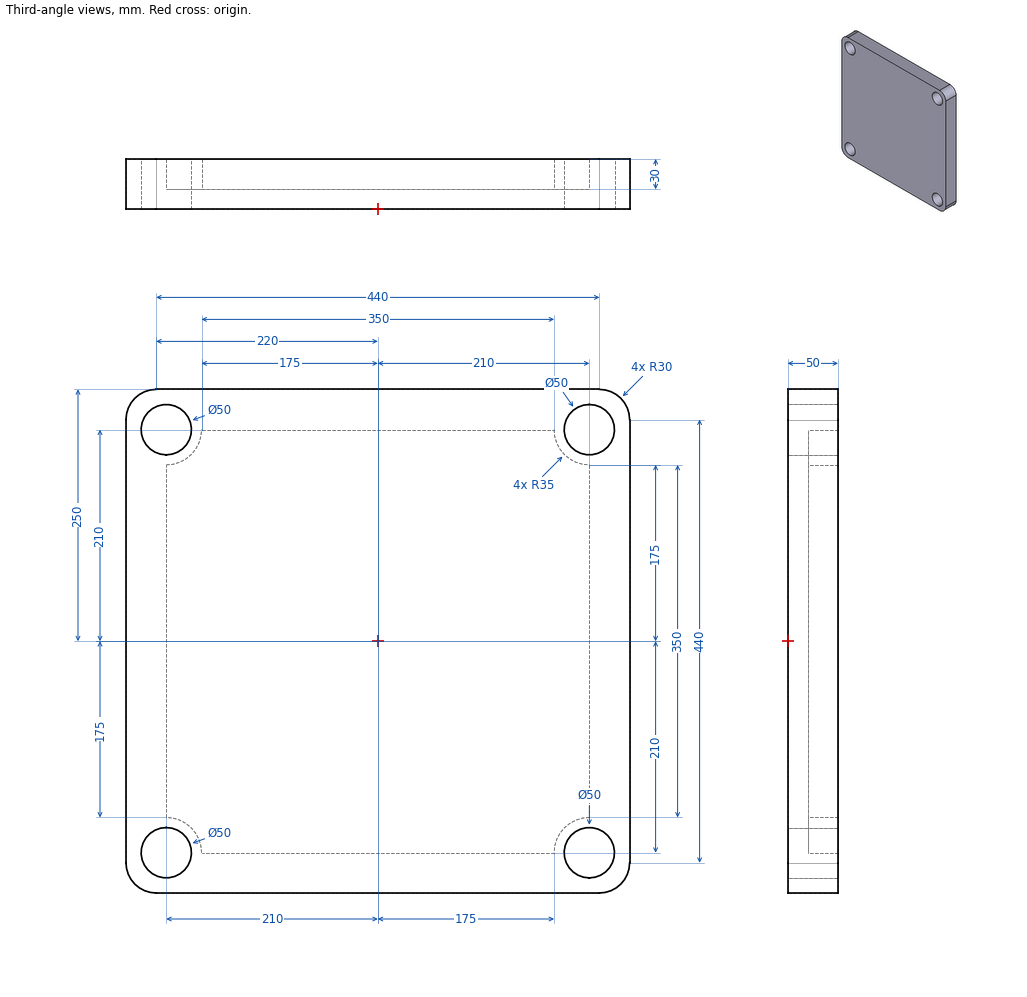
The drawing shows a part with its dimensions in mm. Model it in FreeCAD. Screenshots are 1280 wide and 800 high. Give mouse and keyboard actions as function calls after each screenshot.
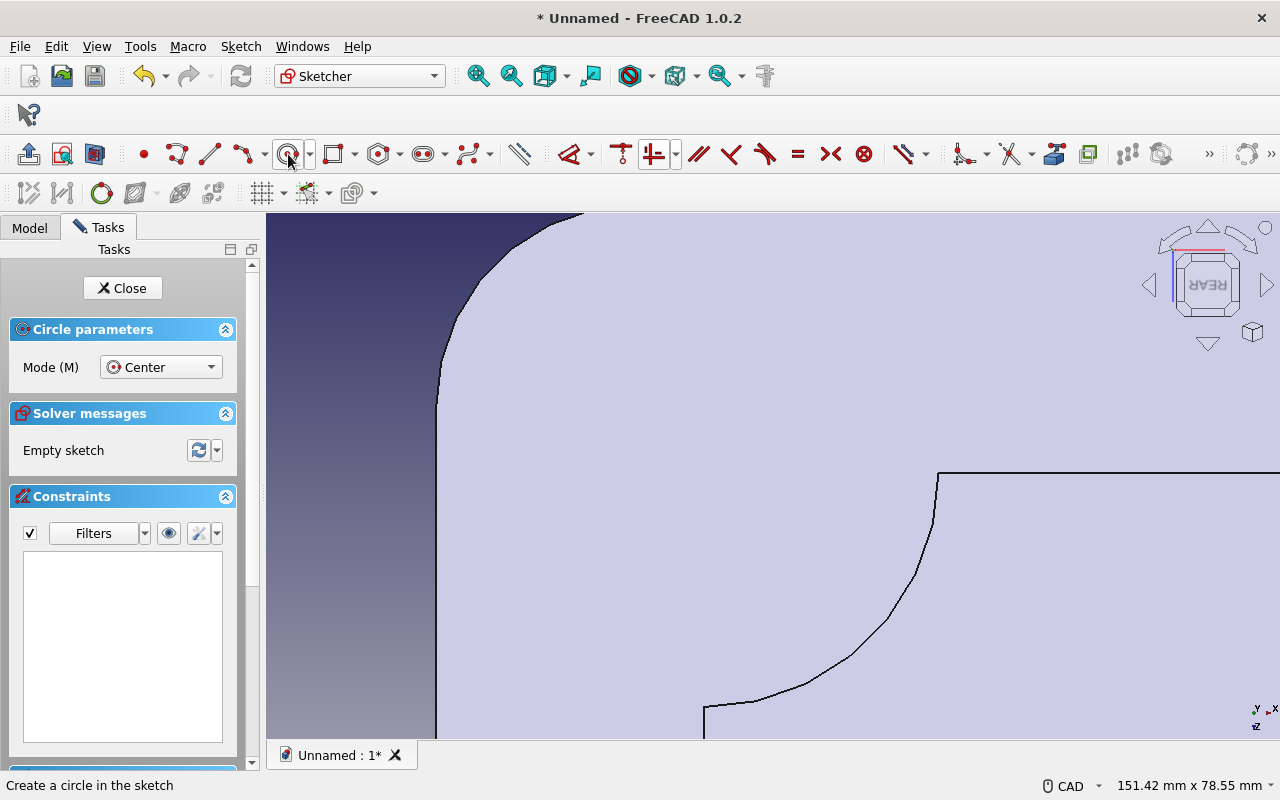
click(704, 473)
move(823, 354)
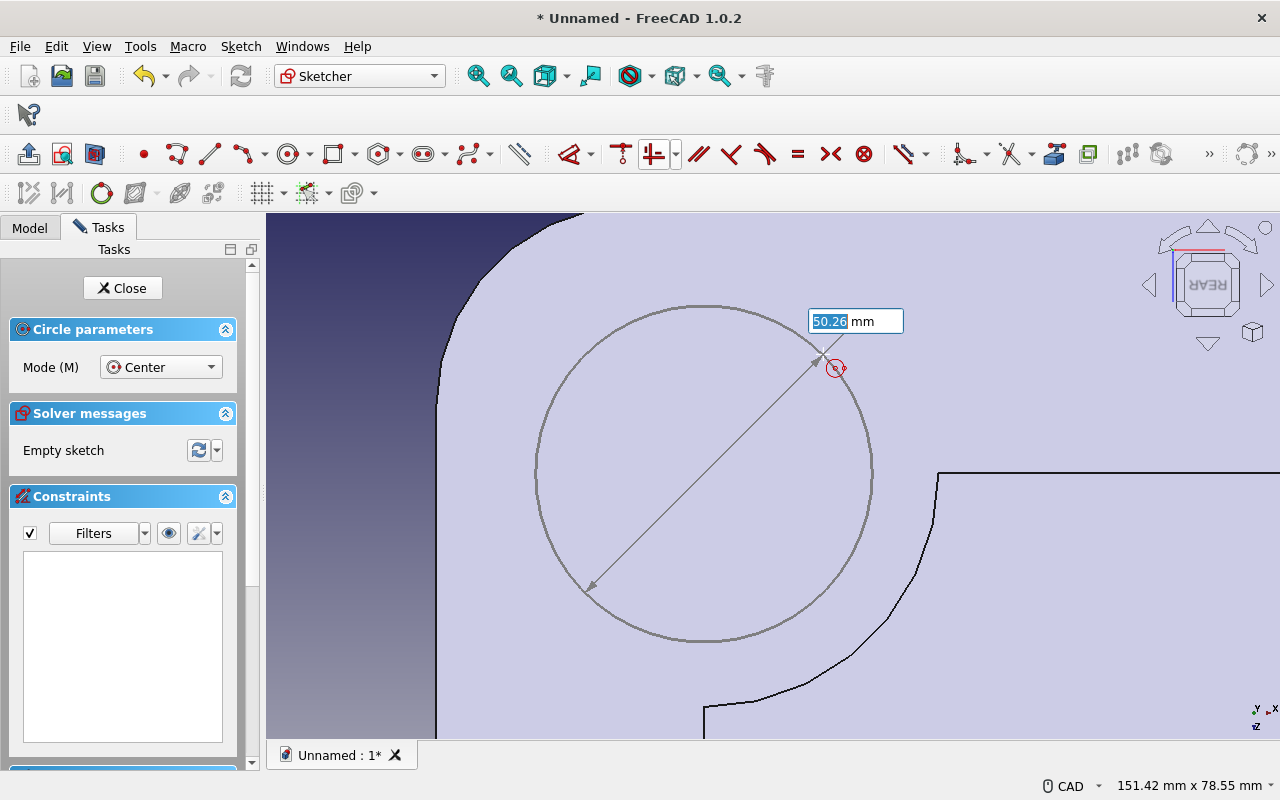
text(50)
key(Return)
key(Escape)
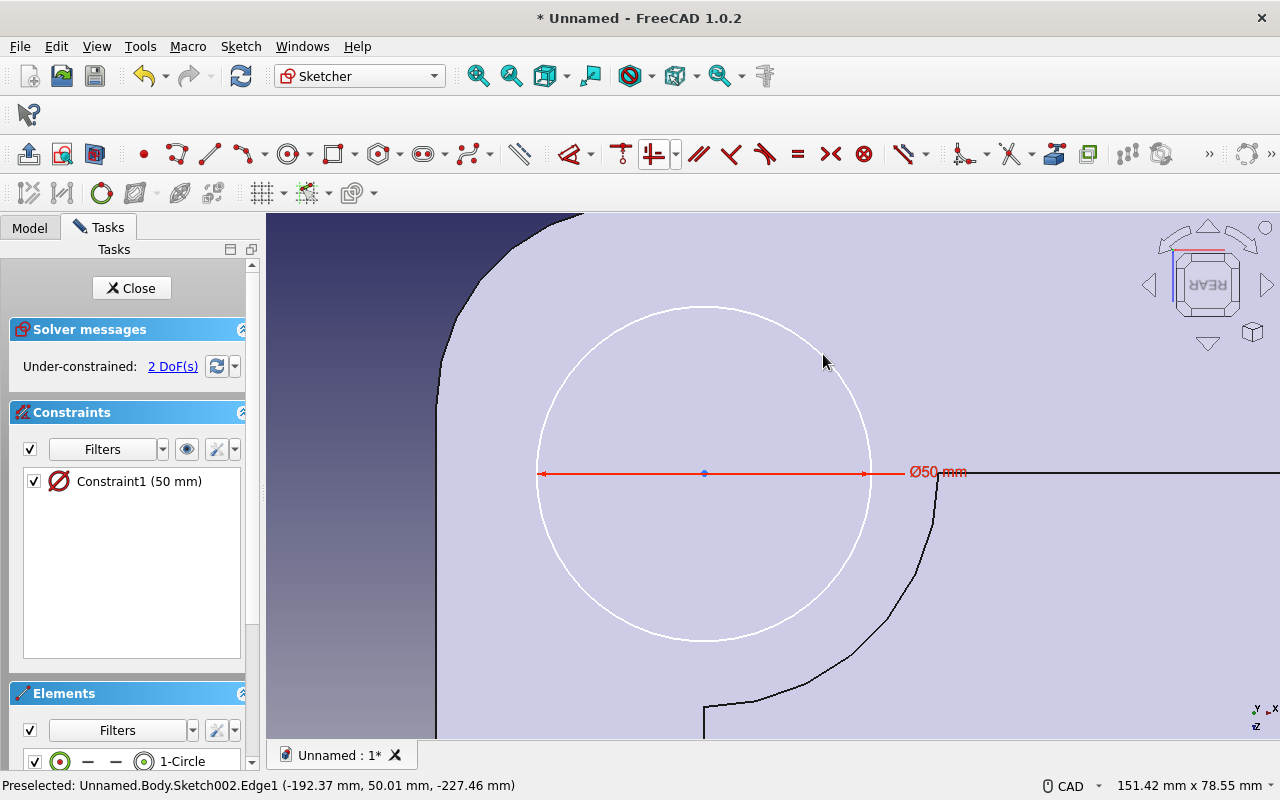
click(568, 154)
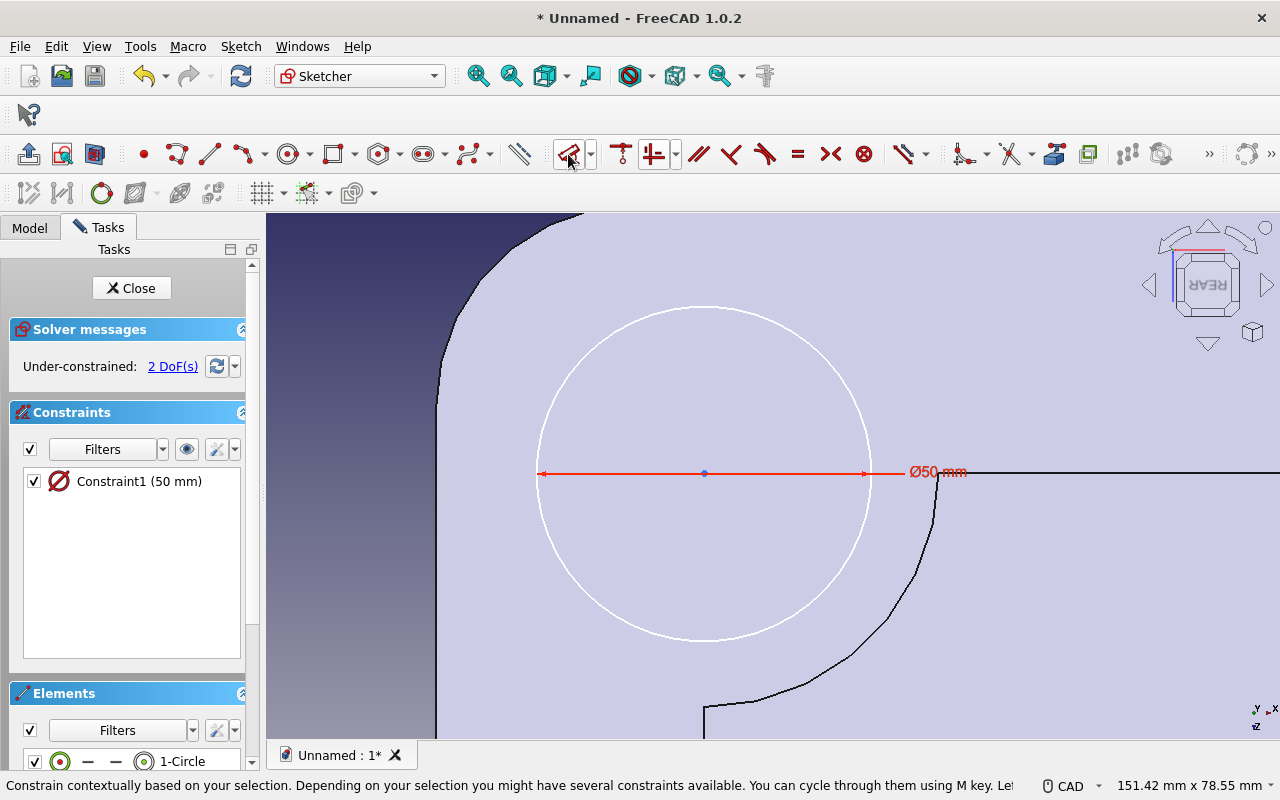
click(704, 474)
click(909, 440)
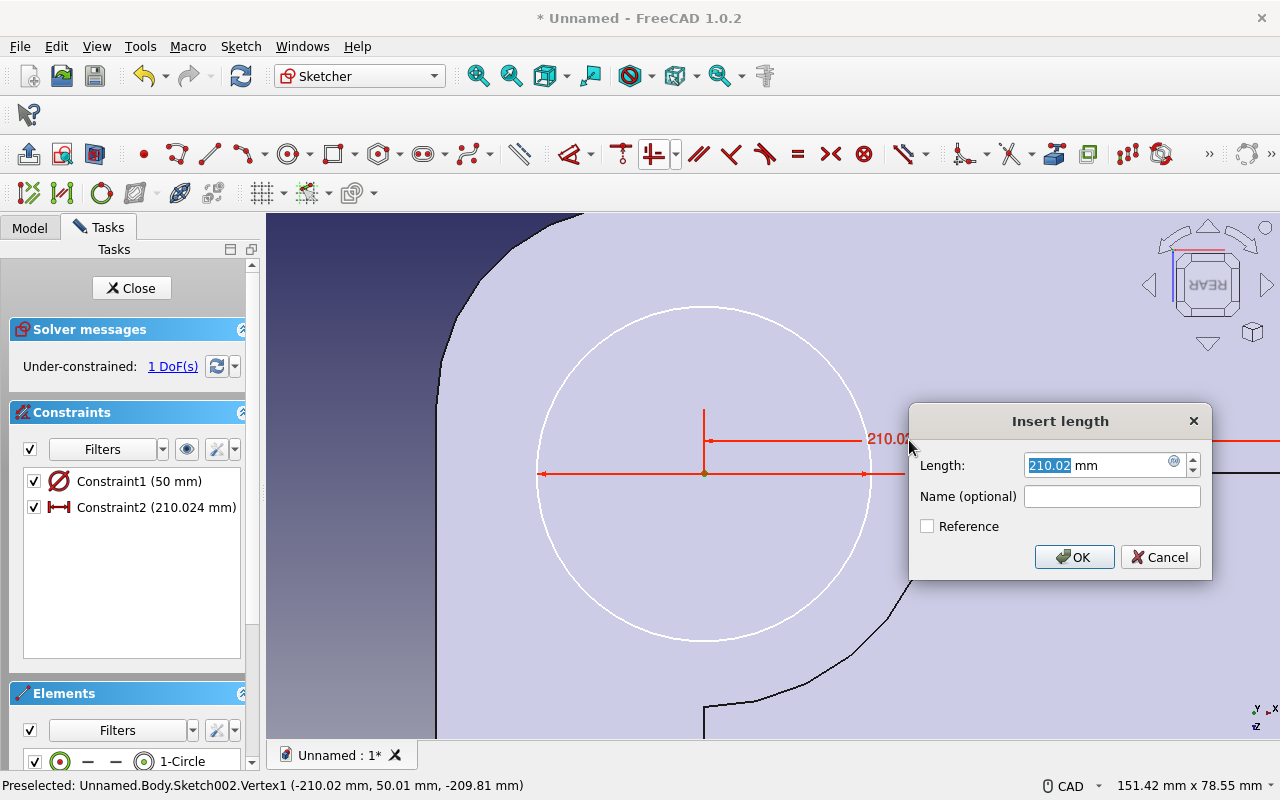
text(210)
key(Return)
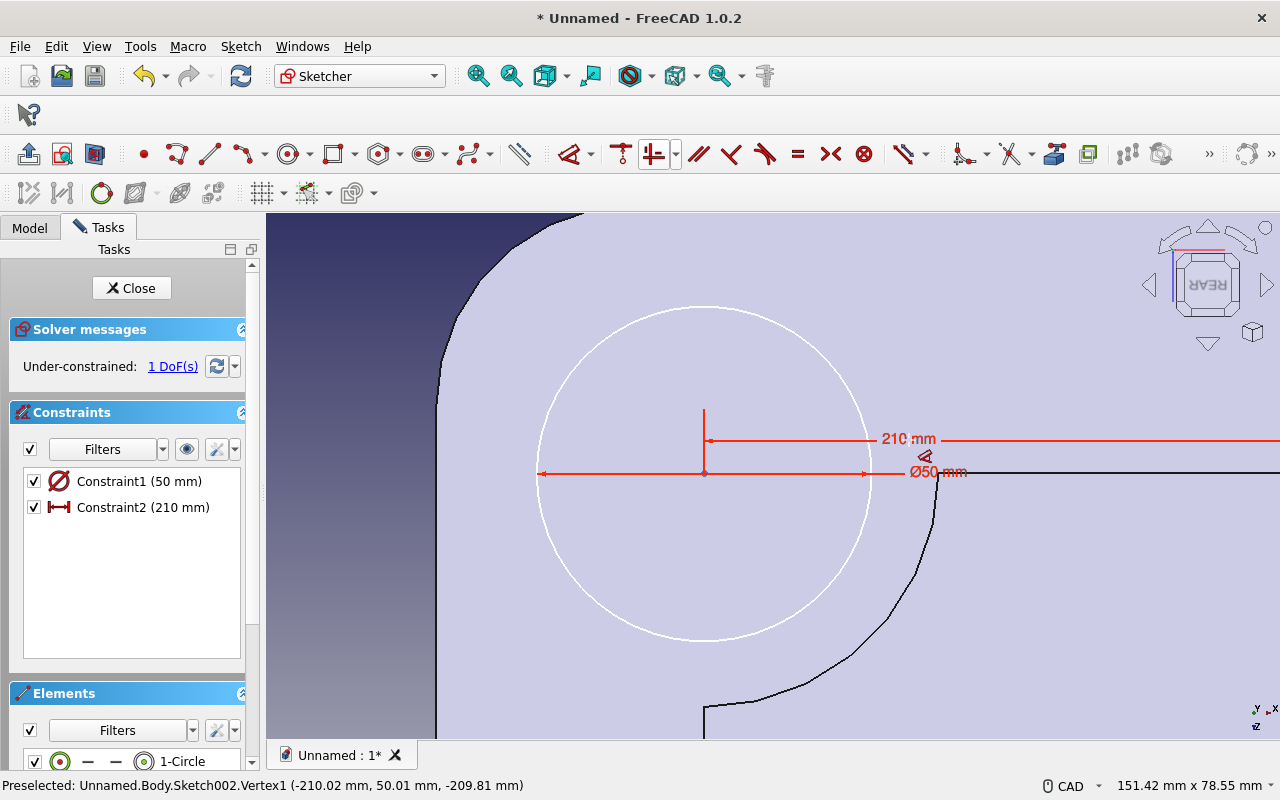
click(704, 474)
click(670, 592)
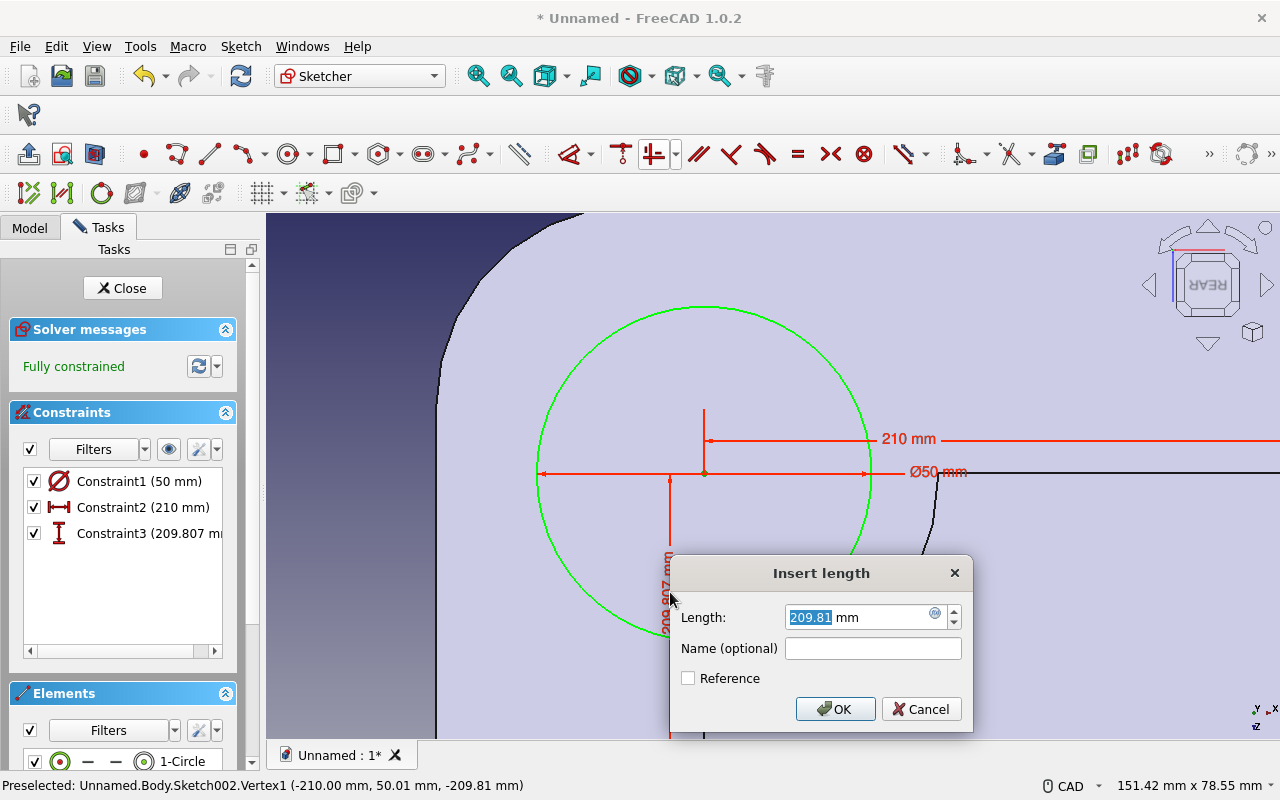
text(210)
key(Return)
key(Escape)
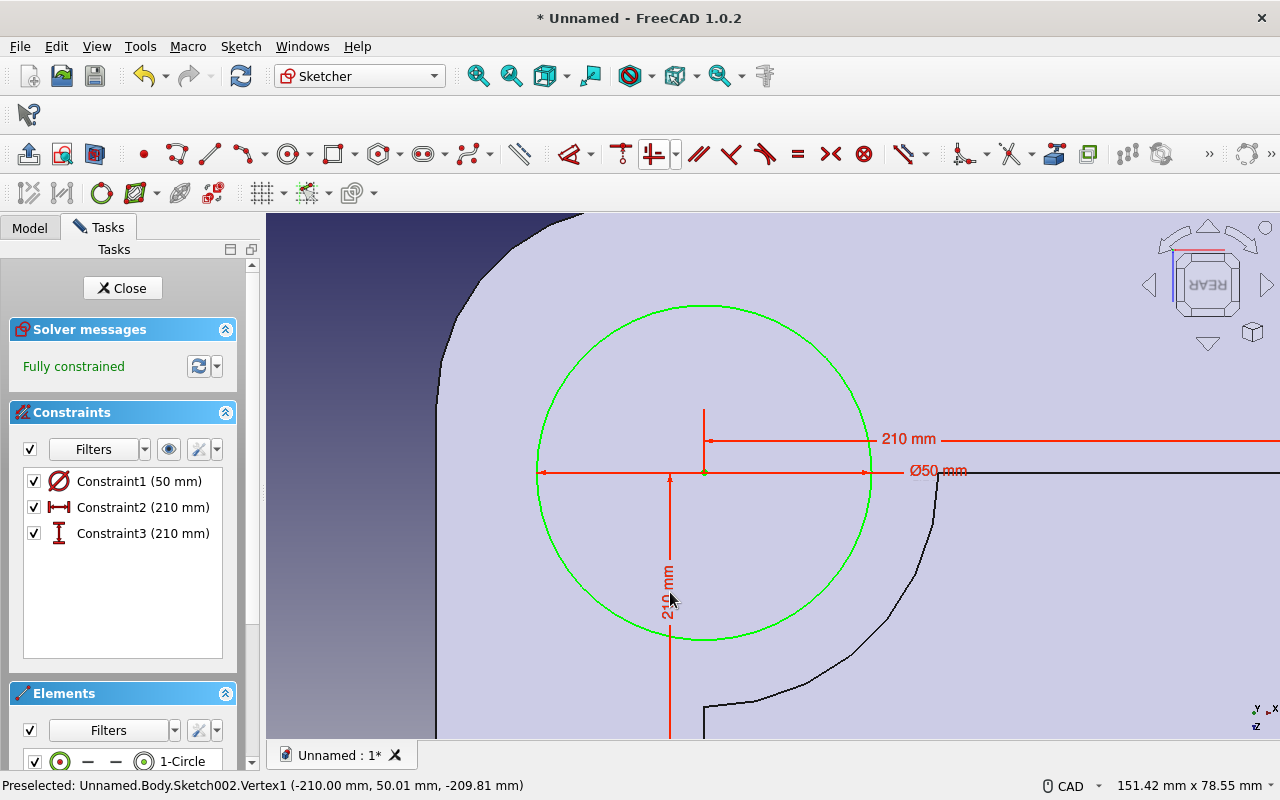
click(123, 288)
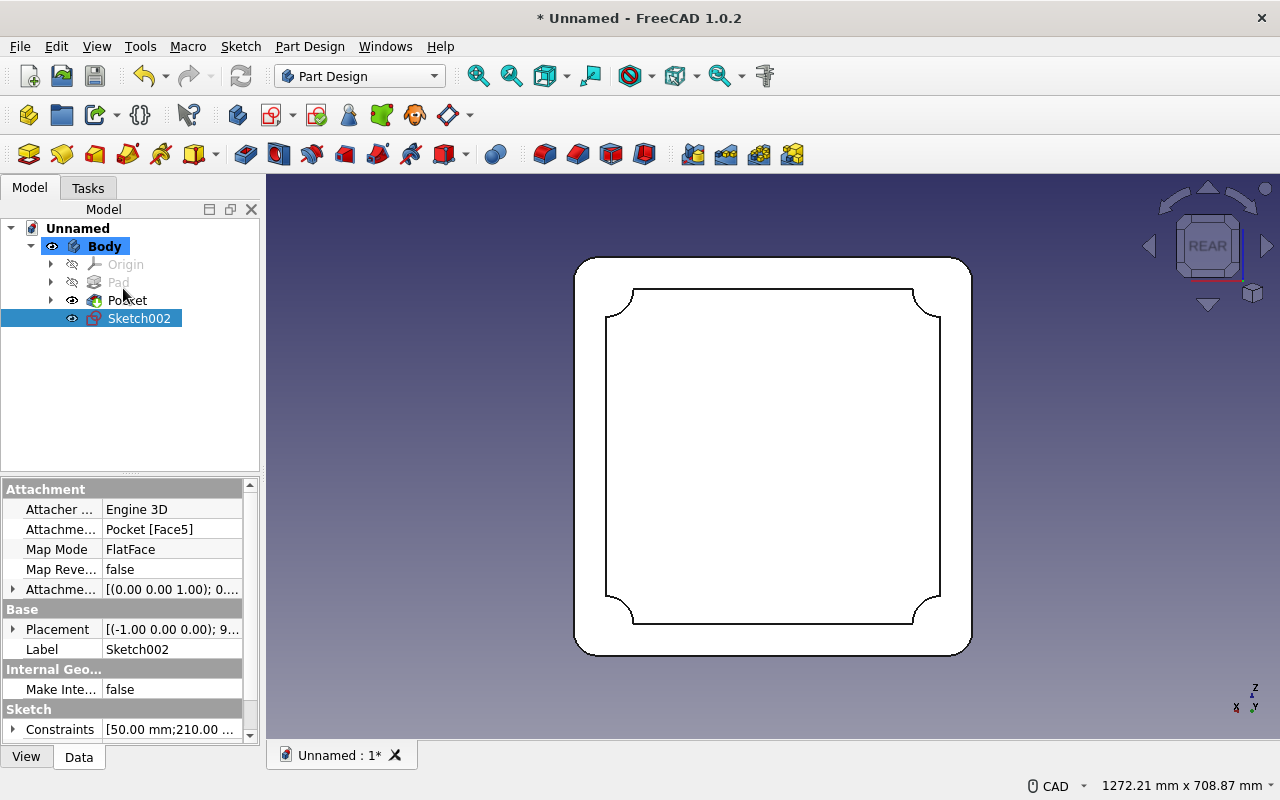
click(246, 154)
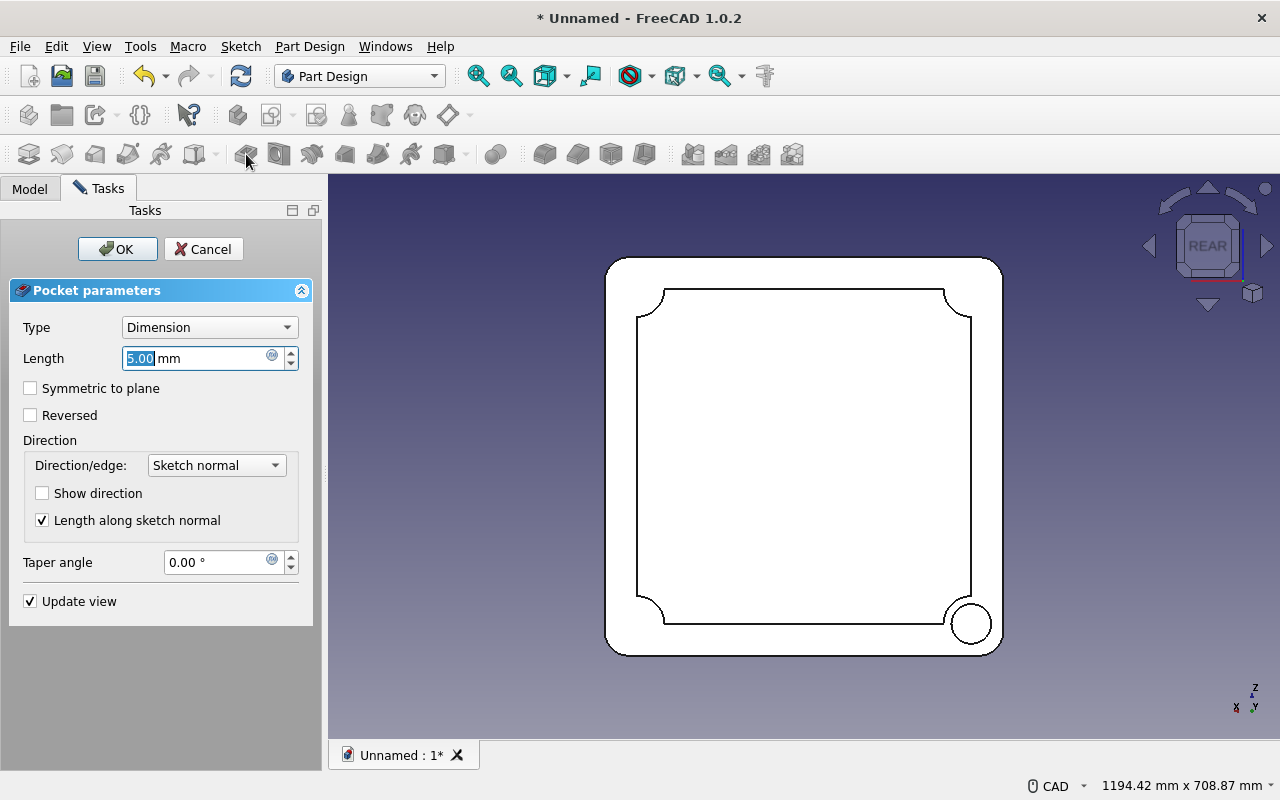
click(210, 328)